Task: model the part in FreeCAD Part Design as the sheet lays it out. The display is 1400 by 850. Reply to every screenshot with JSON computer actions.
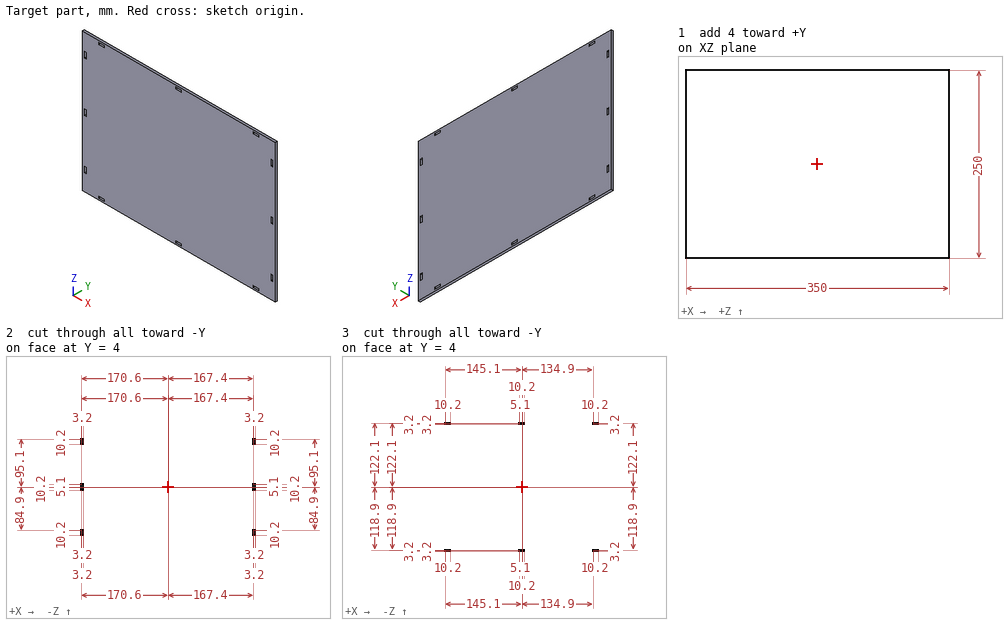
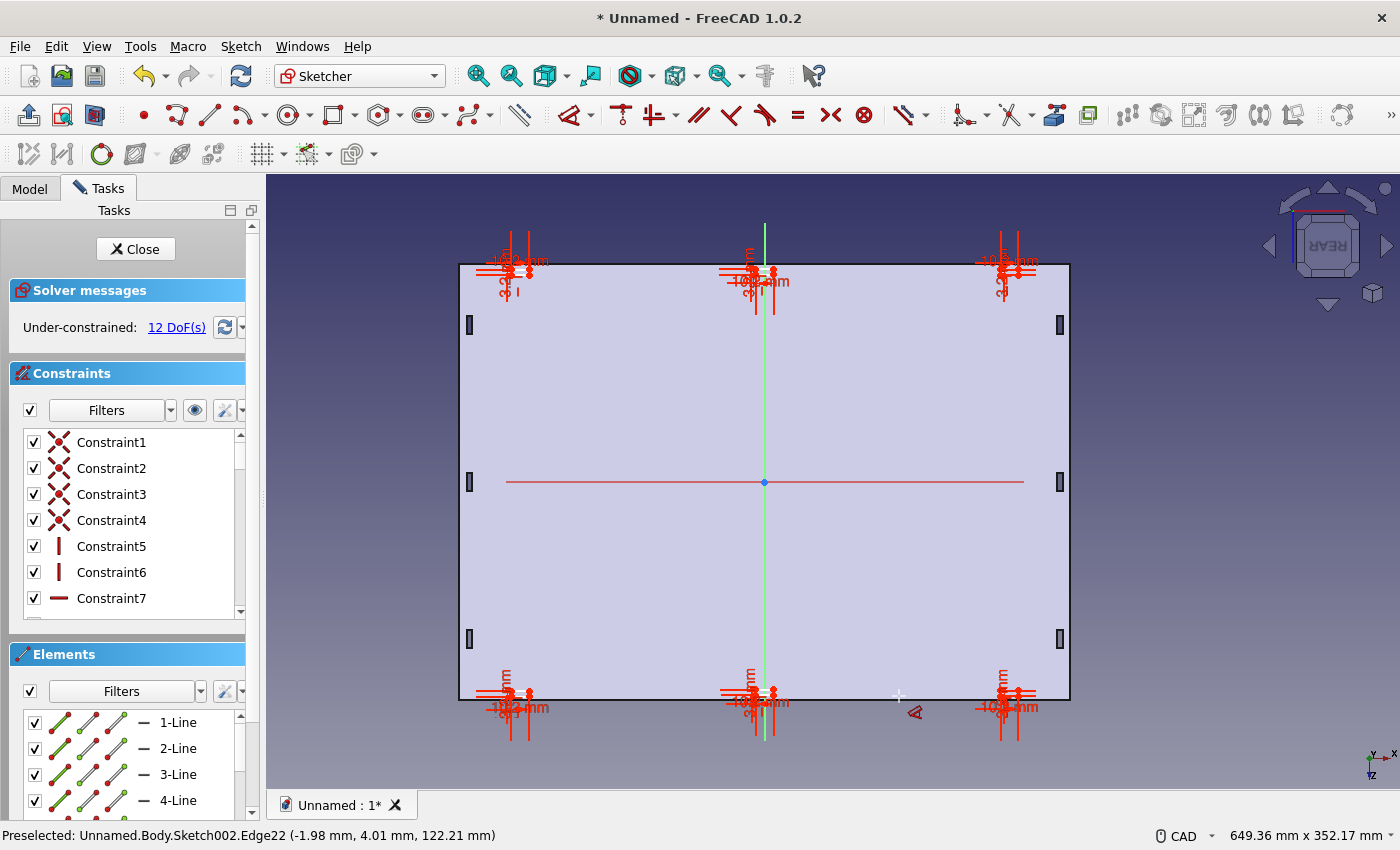
{"action": "scroll", "coordinate": [756, 269], "scroll_direction": "up", "scroll_amount": 8}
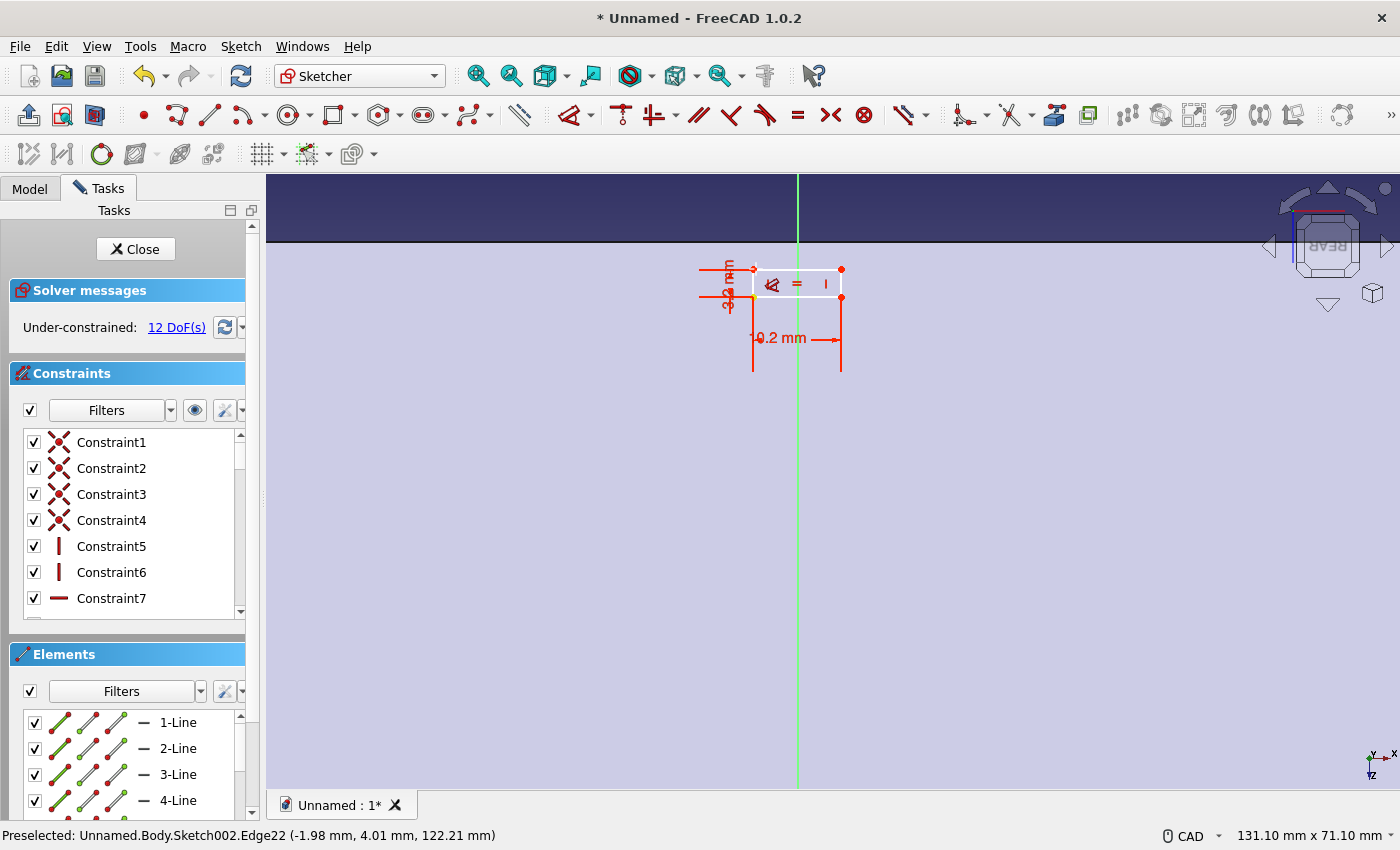
{"action": "left_click", "coordinate": [753, 270]}
{"action": "left_click", "coordinate": [775, 236]}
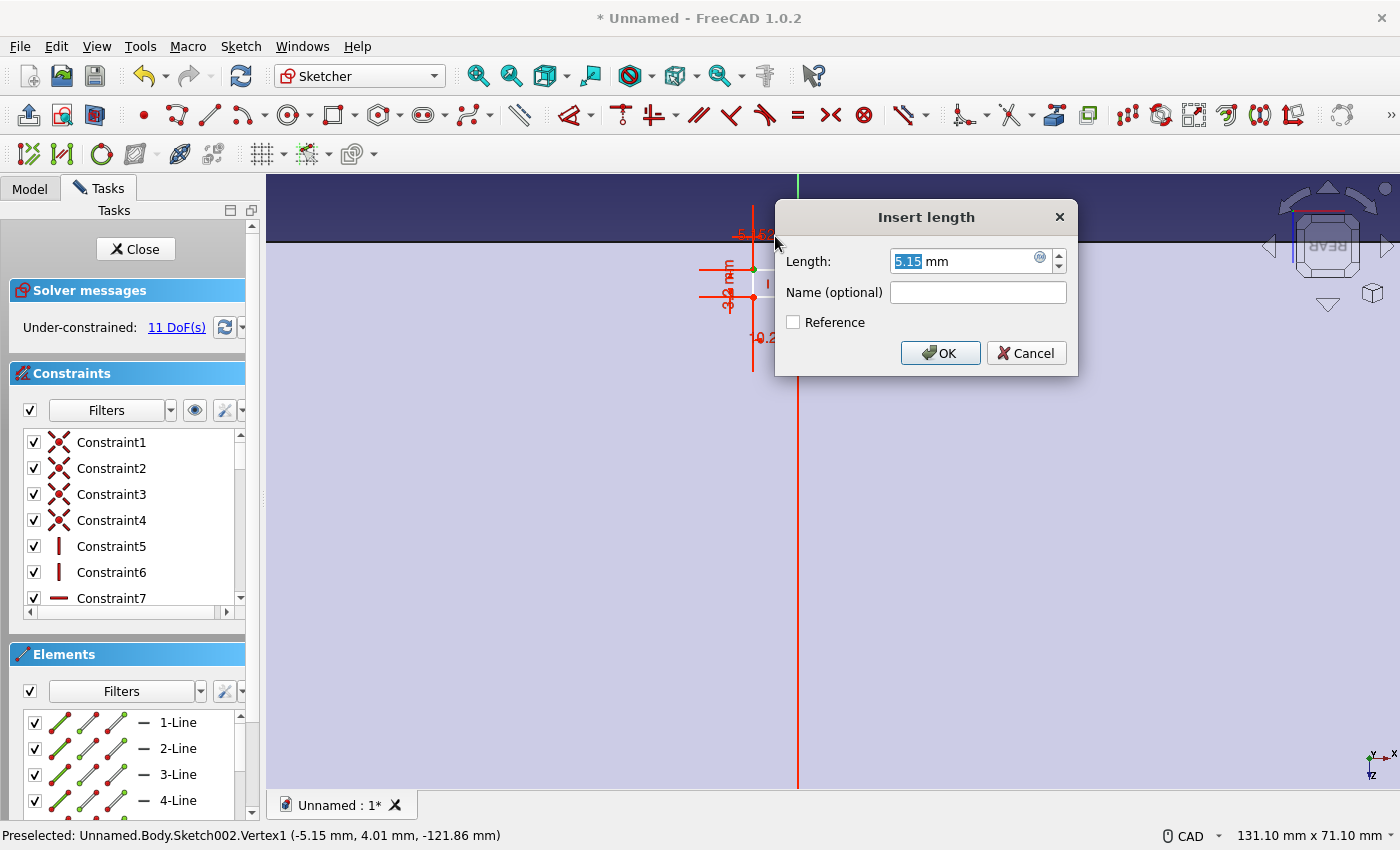
{"action": "type", "text": "5.1"}
{"action": "key", "text": "Return"}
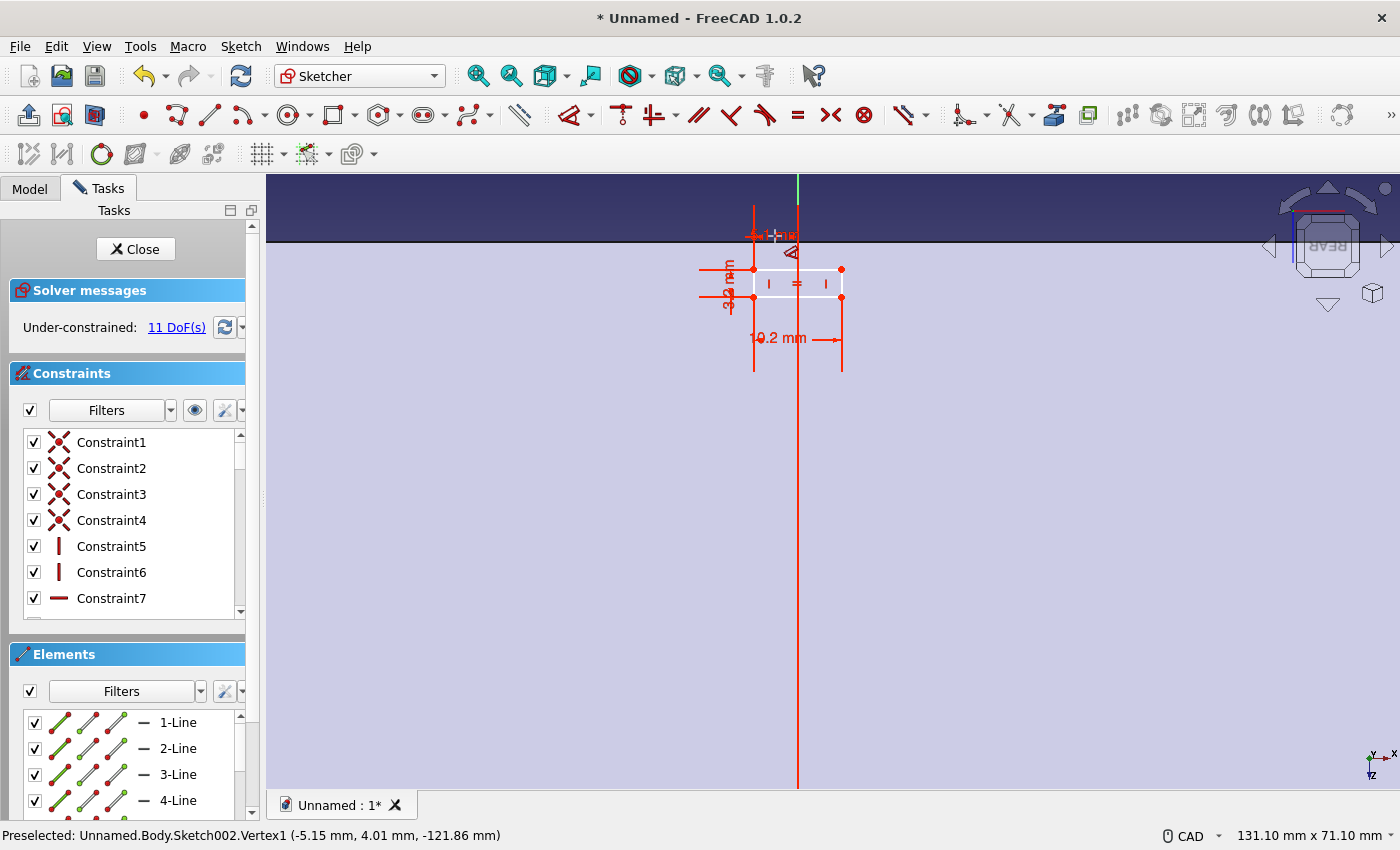
{"action": "scroll", "coordinate": [756, 268], "scroll_direction": "down", "scroll_amount": 8}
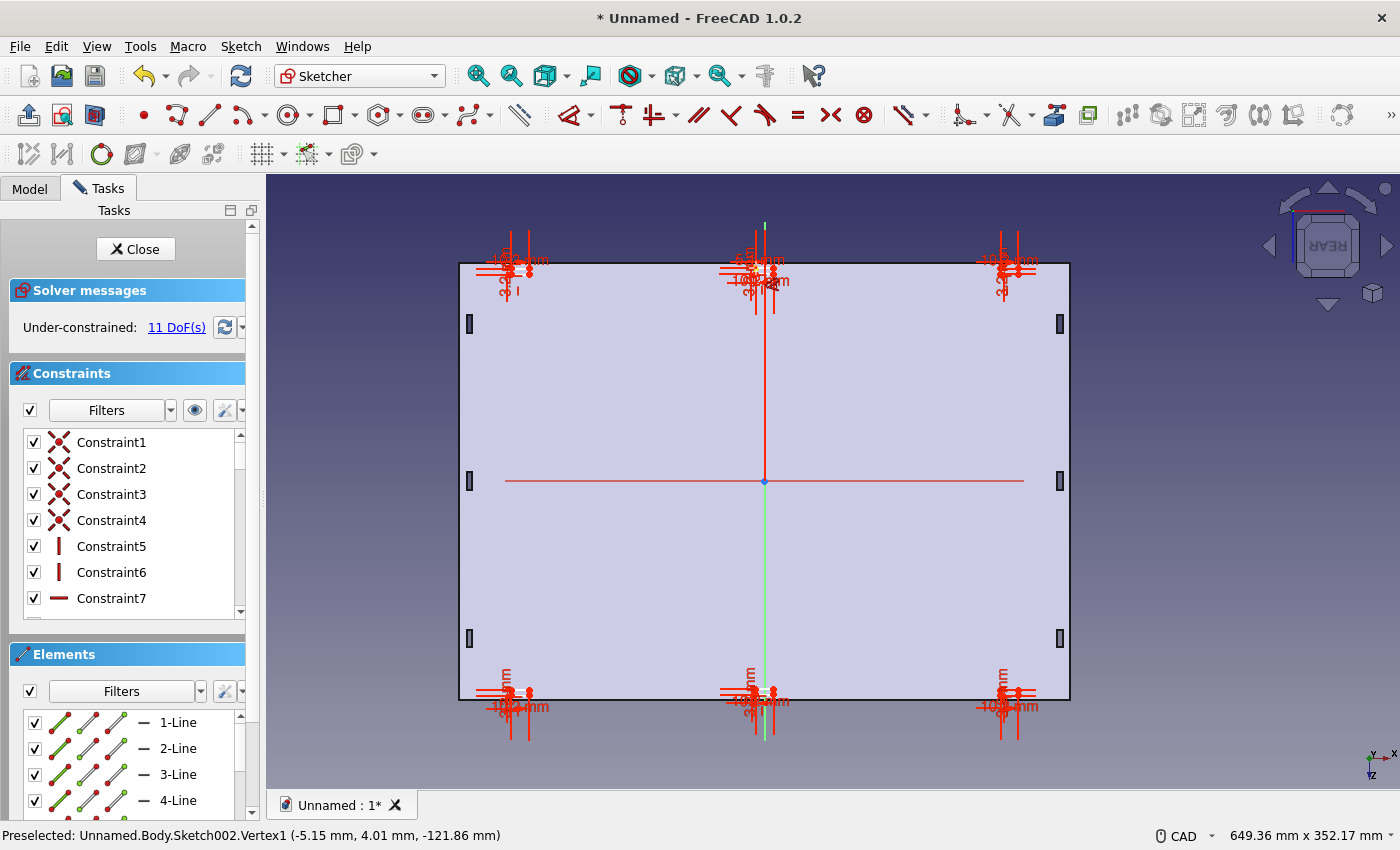
{"action": "scroll", "coordinate": [756, 689], "scroll_direction": "up", "scroll_amount": 8}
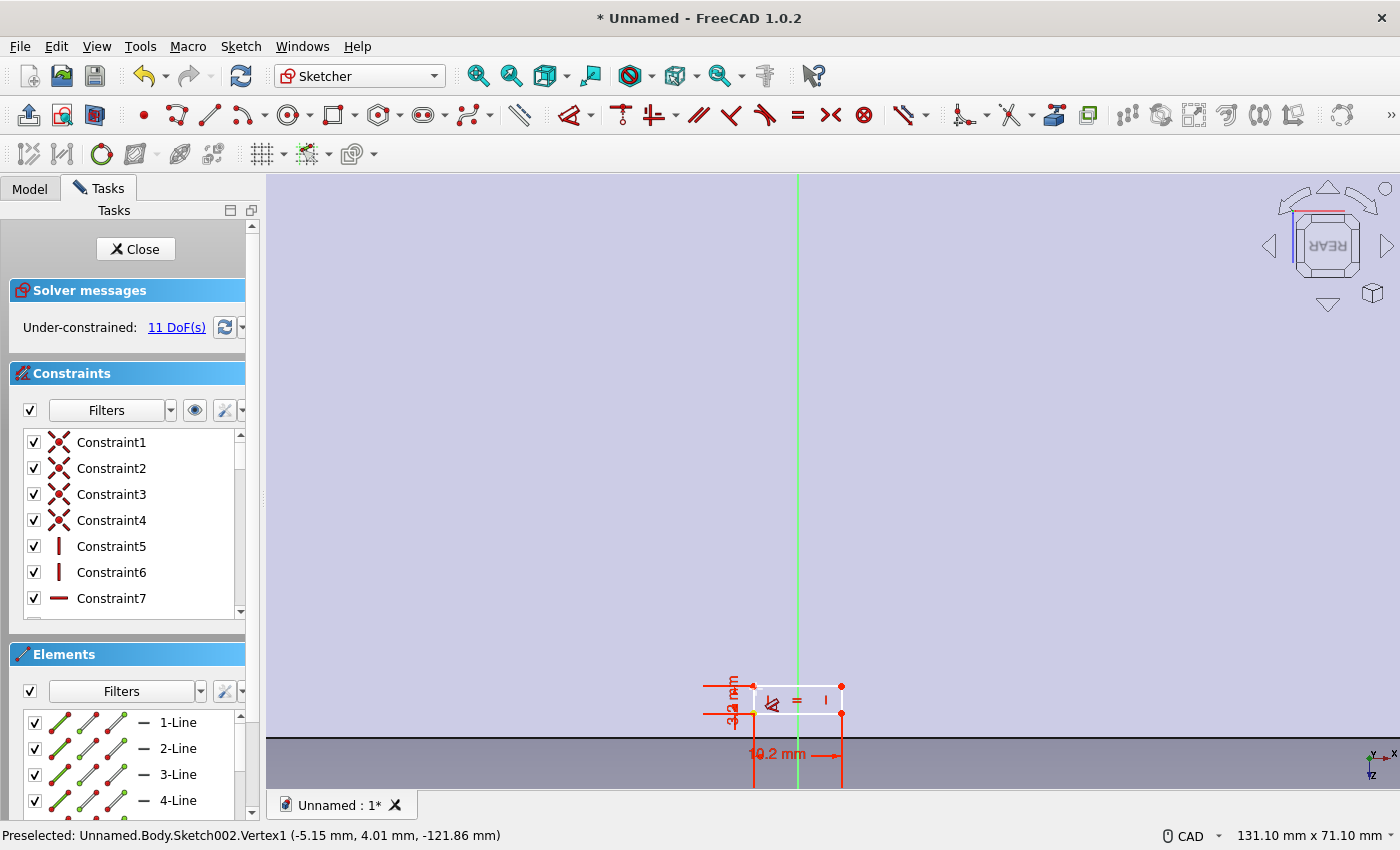
{"action": "left_click", "coordinate": [754, 686]}
{"action": "left_click", "coordinate": [776, 744]}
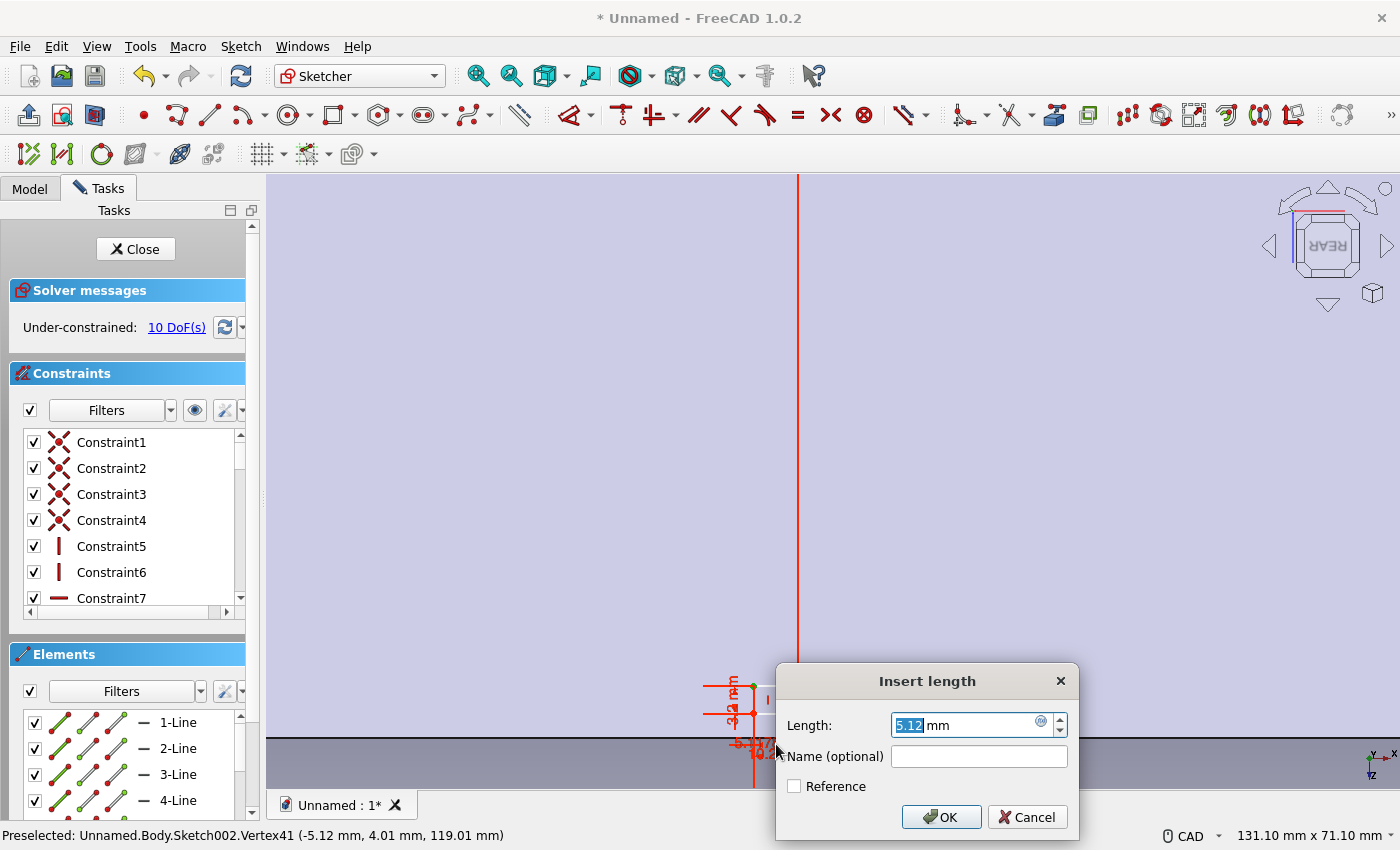
{"action": "type", "text": "5.1"}
{"action": "key", "text": "Return"}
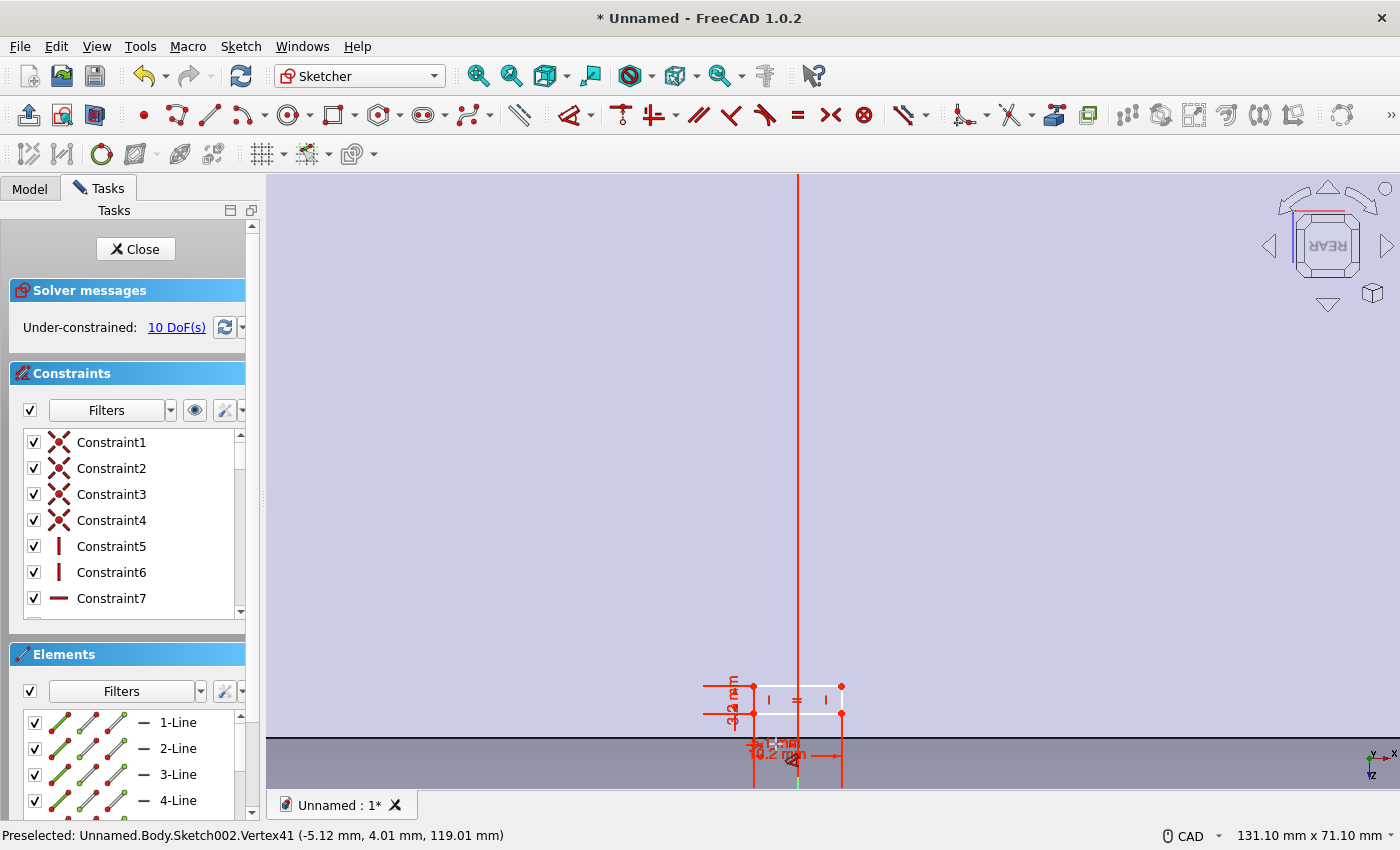
{"action": "scroll", "coordinate": [756, 690], "scroll_direction": "down", "scroll_amount": 8}